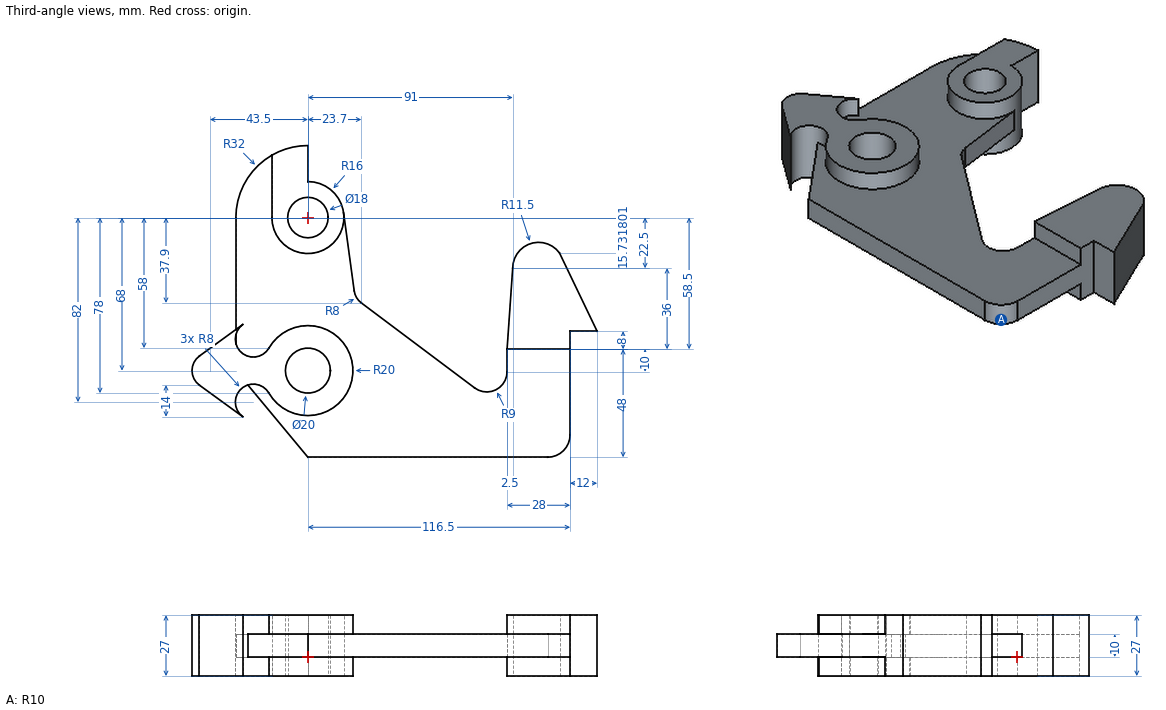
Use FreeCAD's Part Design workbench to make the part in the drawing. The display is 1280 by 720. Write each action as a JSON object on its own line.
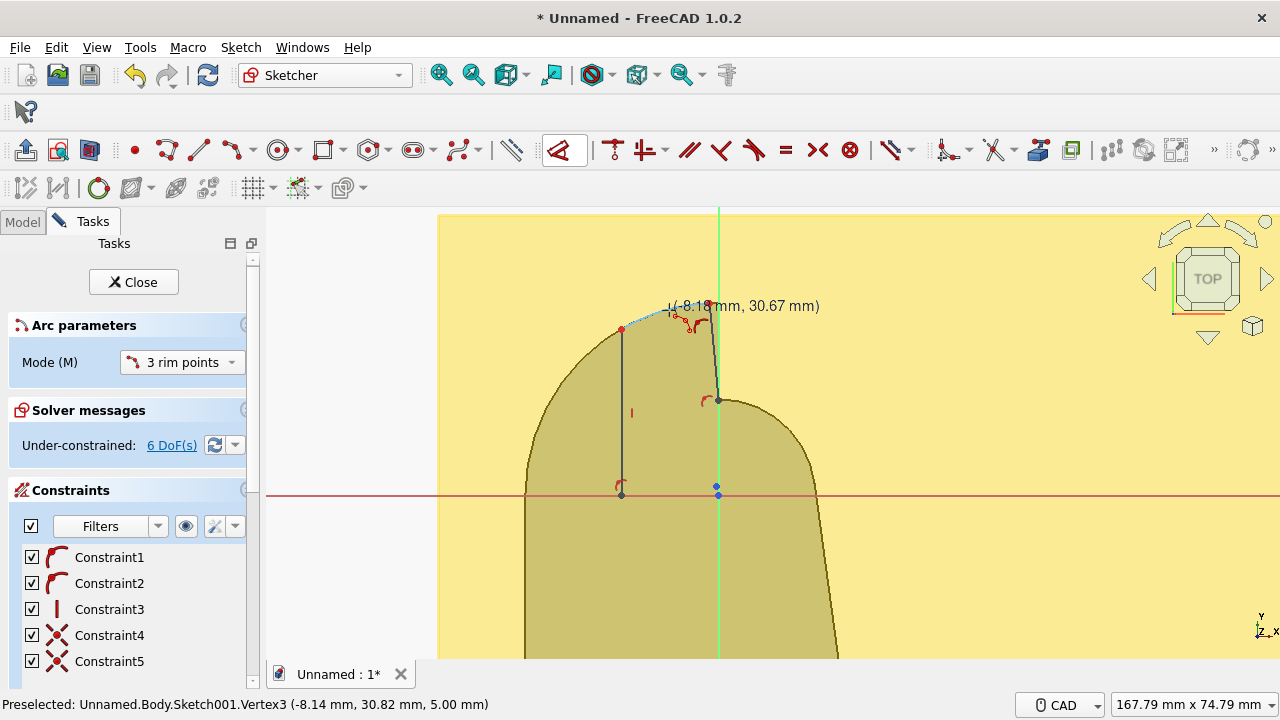
{"action": "left_click", "coordinate": [622, 496]}
{"action": "left_click", "coordinate": [719, 400]}
{"action": "left_click", "coordinate": [787, 564]}
{"action": "key", "text": "Escape"}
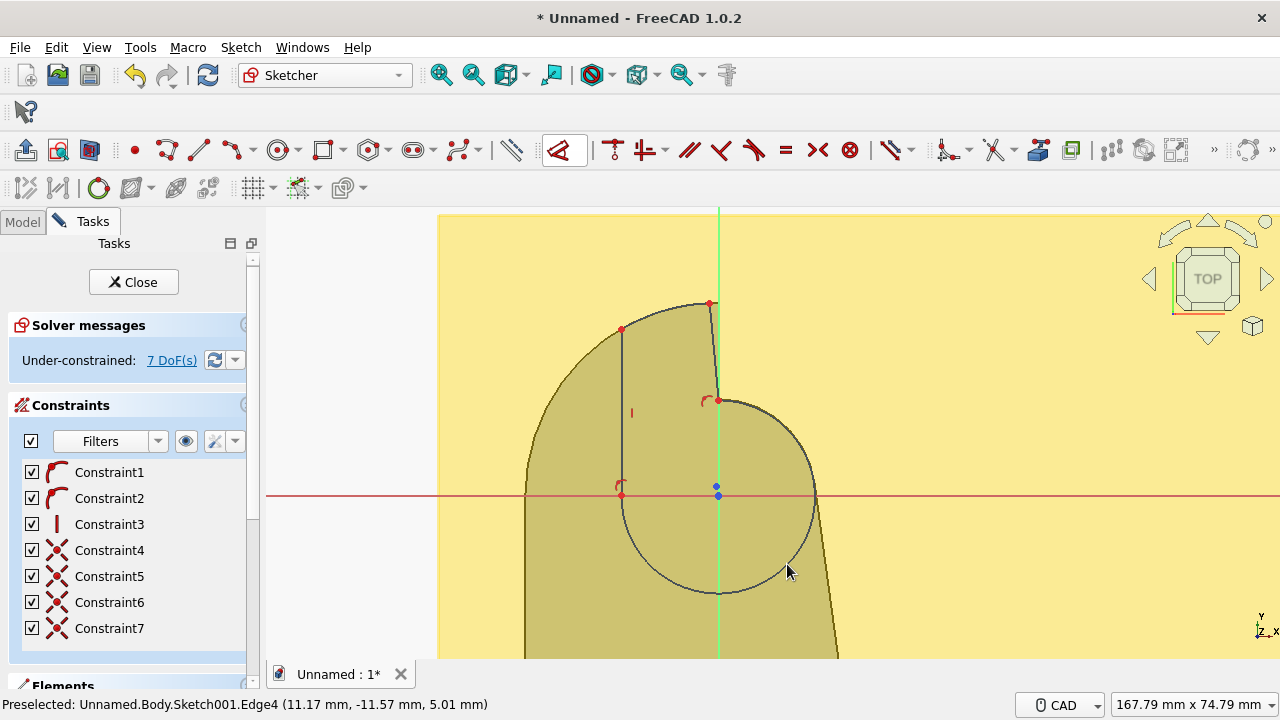
{"action": "left_click", "coordinate": [622, 379]}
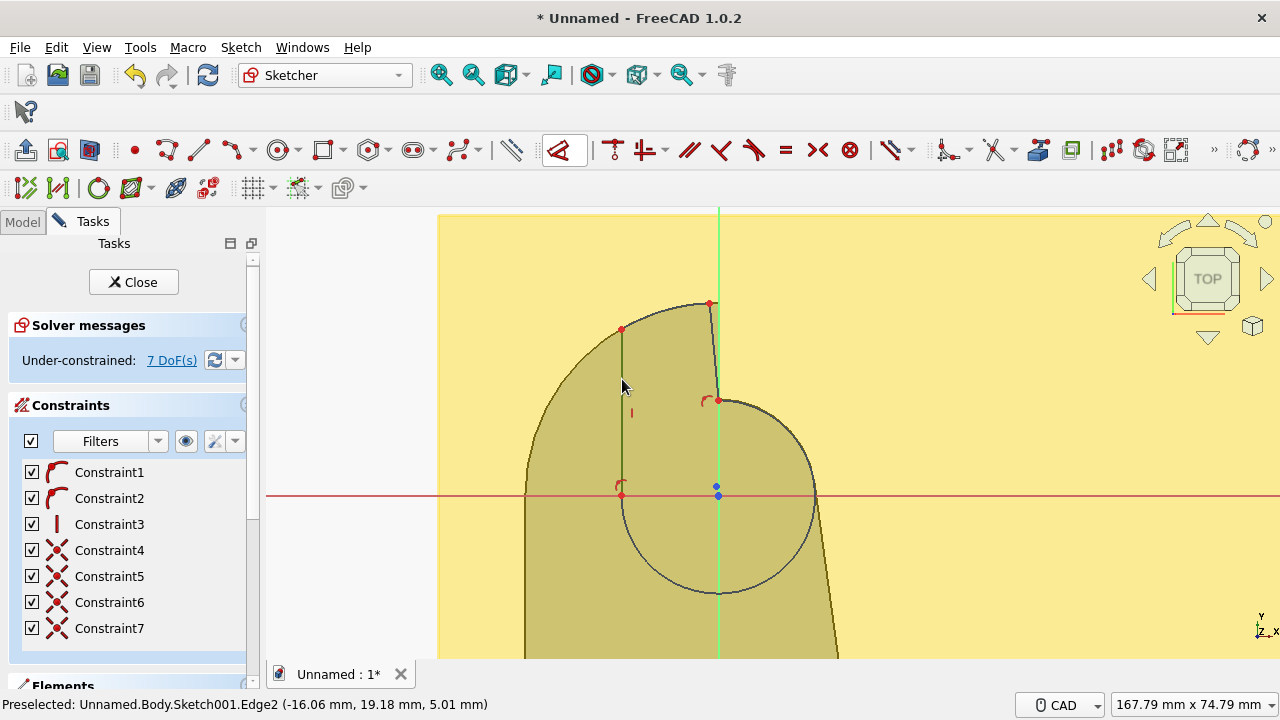
{"action": "left_click", "coordinate": [702, 592]}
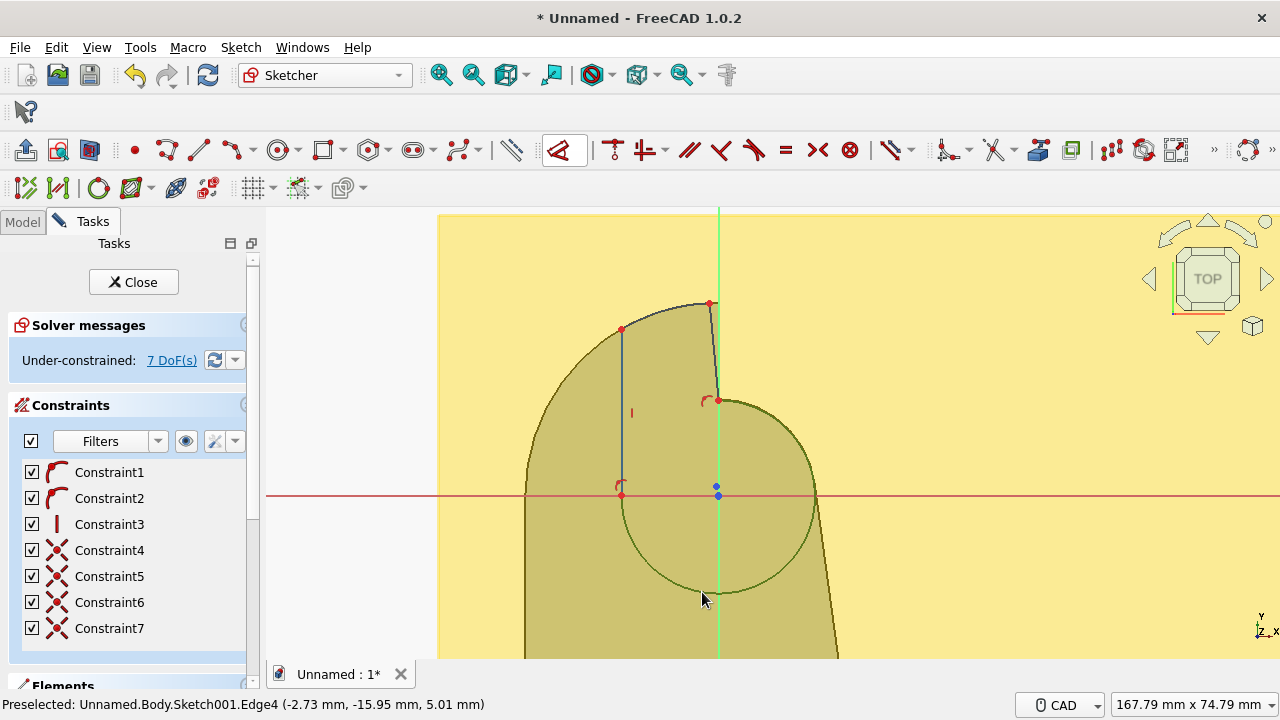
{"action": "left_click", "coordinate": [754, 150]}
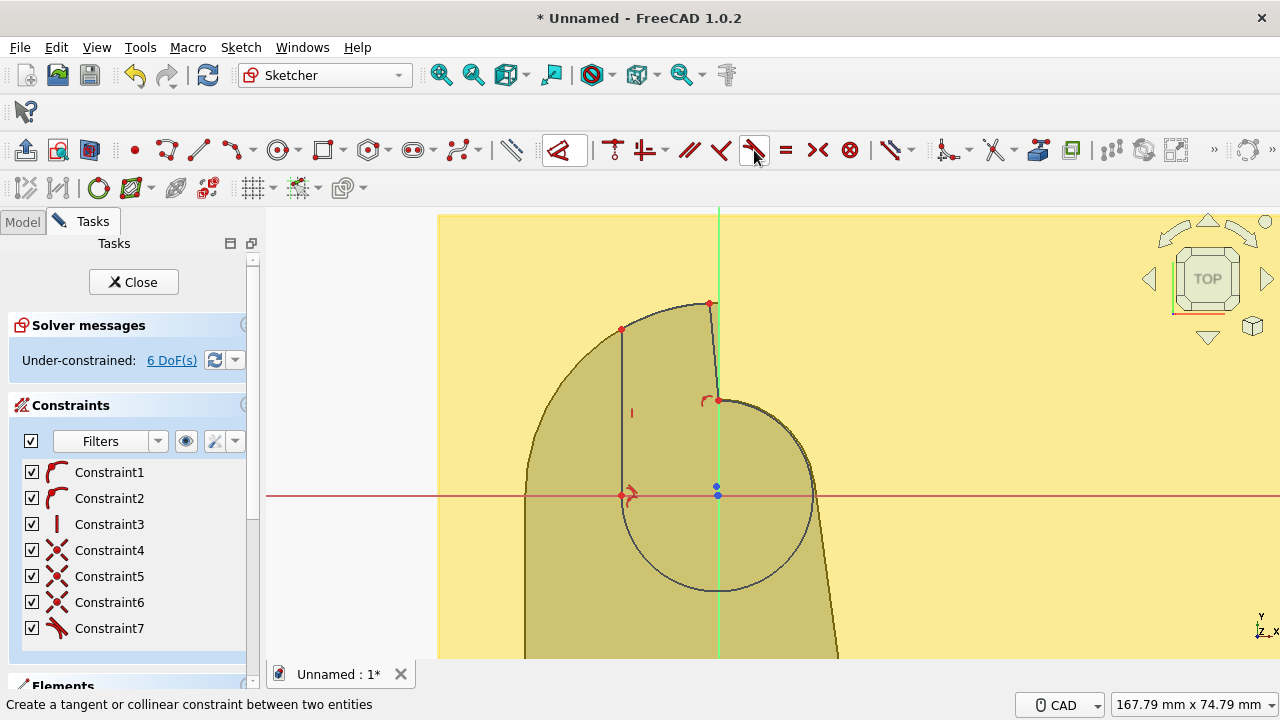
{"action": "left_click", "coordinate": [716, 371]}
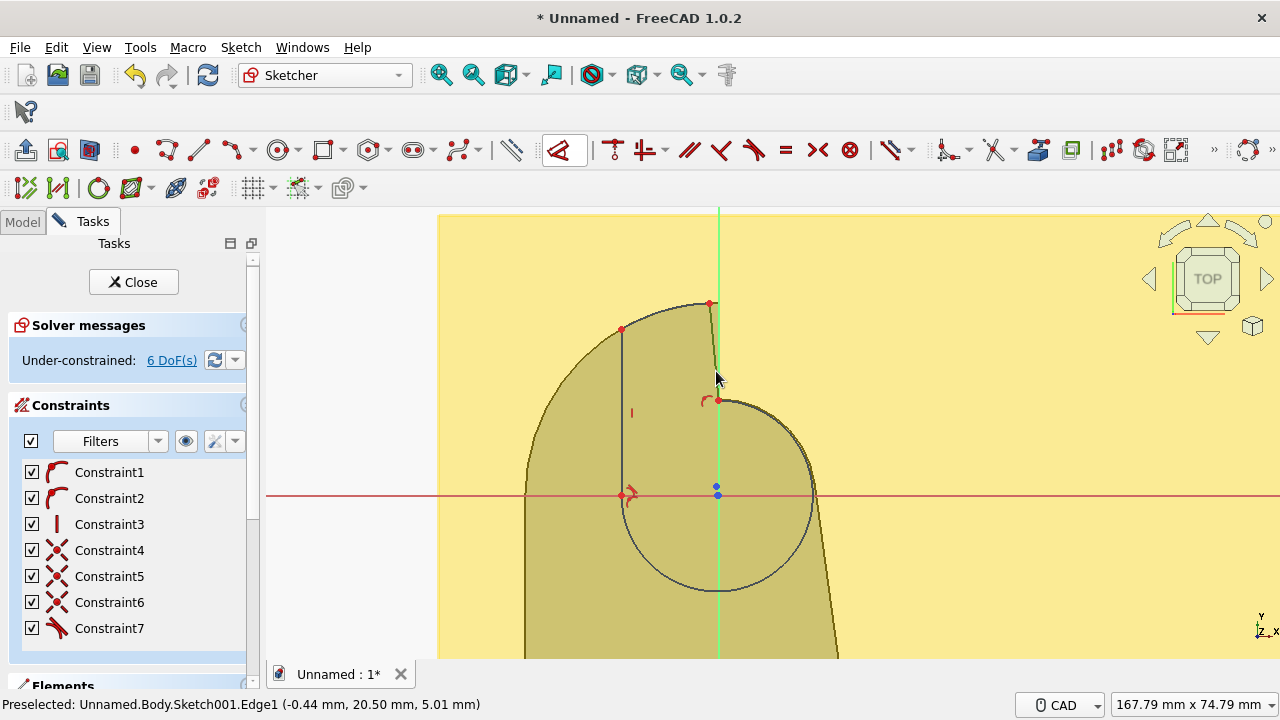
{"action": "left_click", "coordinate": [668, 150]}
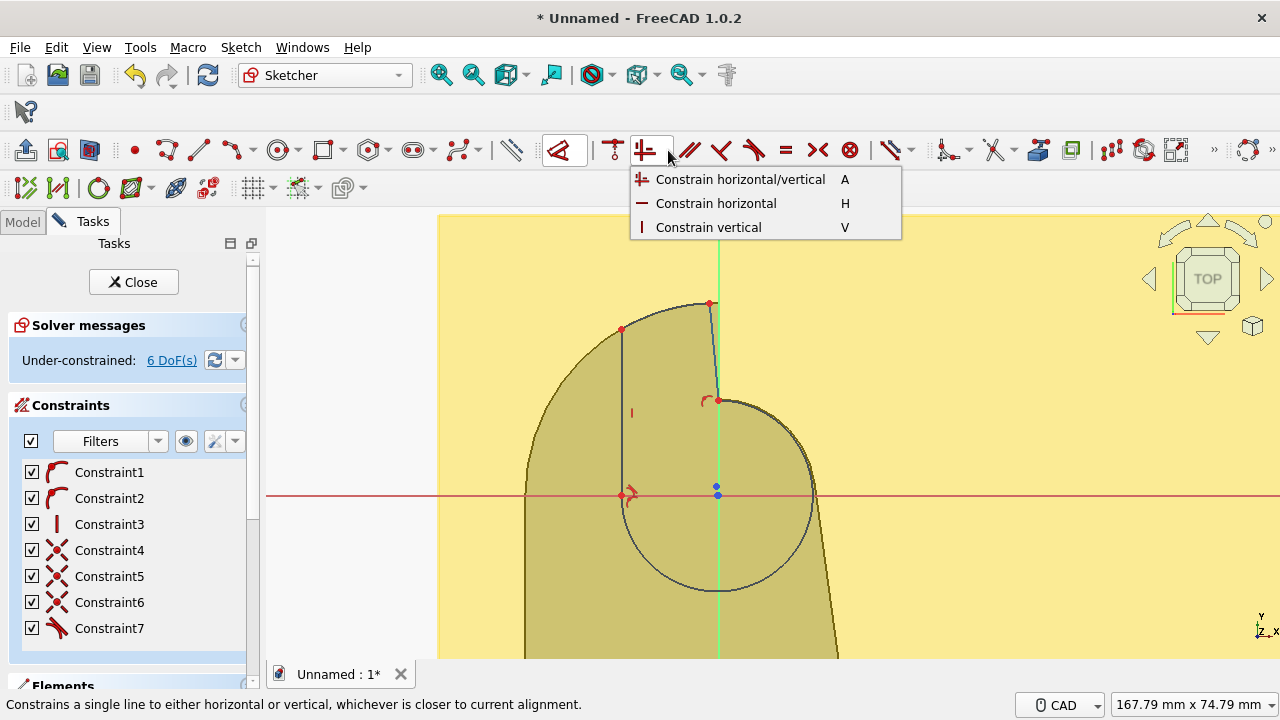
{"action": "left_click", "coordinate": [766, 227]}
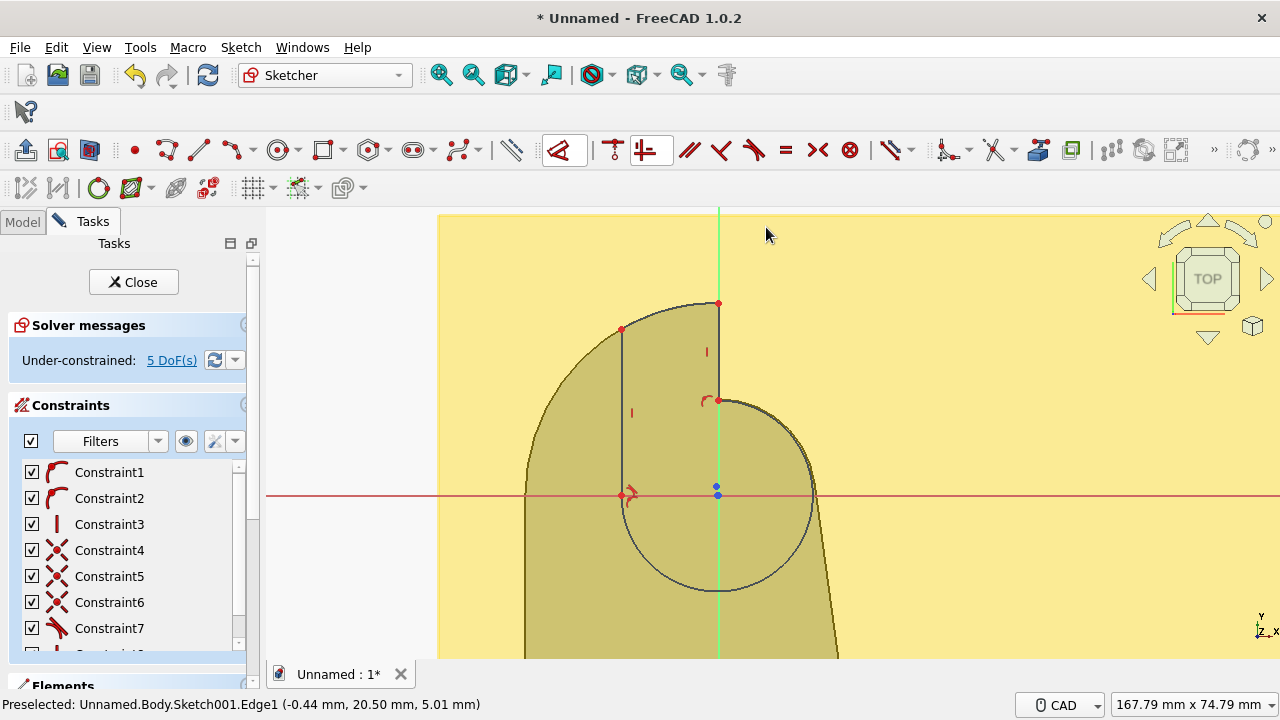
{"action": "left_click", "coordinate": [688, 305]}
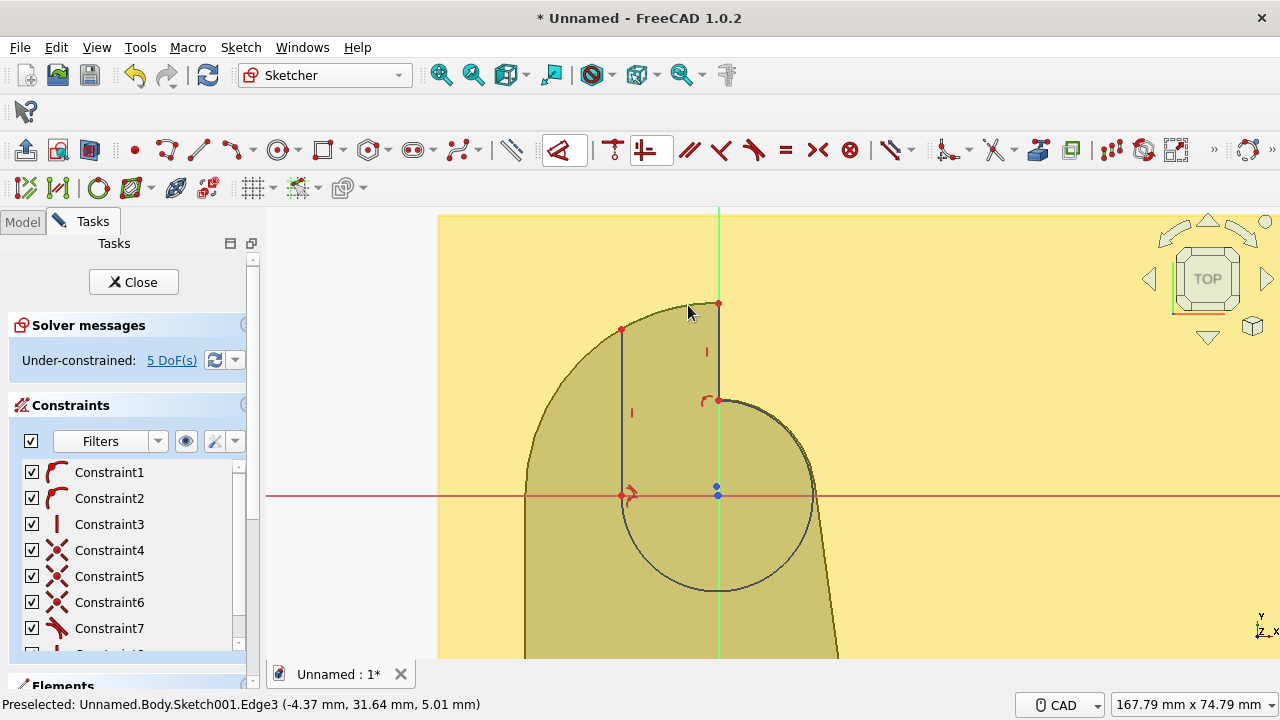
{"action": "left_click", "coordinate": [702, 590]}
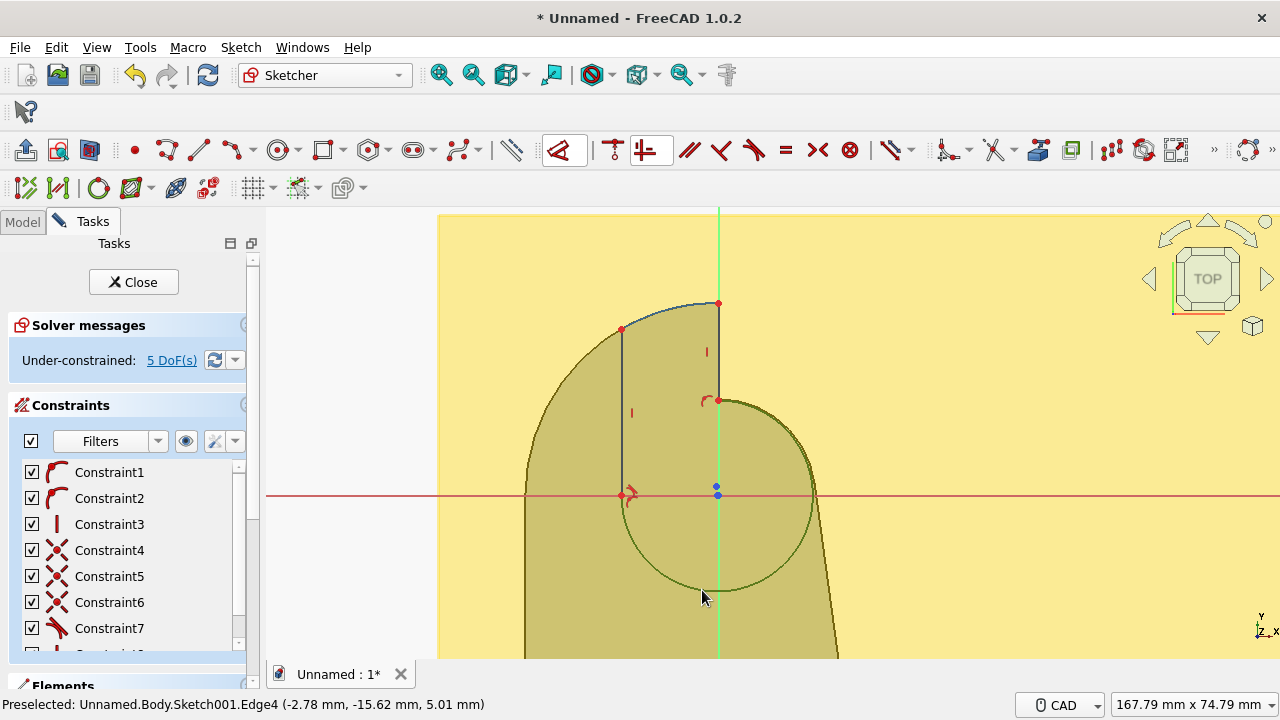
{"action": "left_click", "coordinate": [614, 150]}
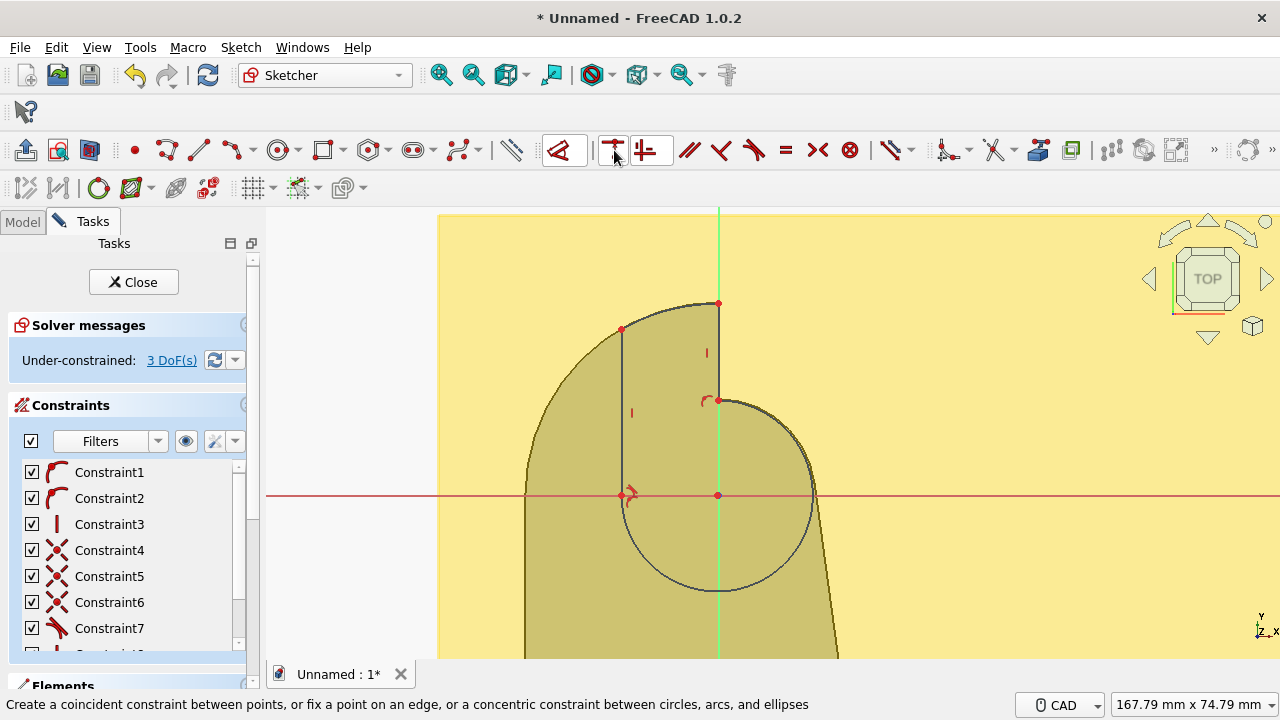
{"action": "left_click", "coordinate": [717, 496]}